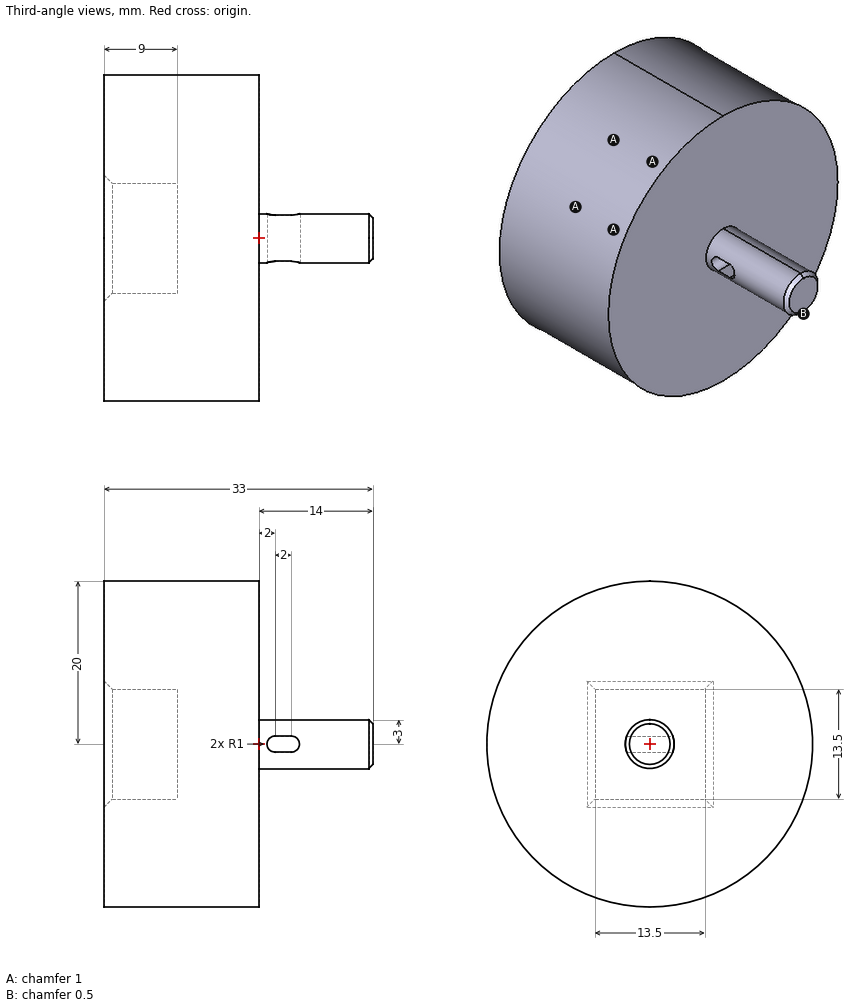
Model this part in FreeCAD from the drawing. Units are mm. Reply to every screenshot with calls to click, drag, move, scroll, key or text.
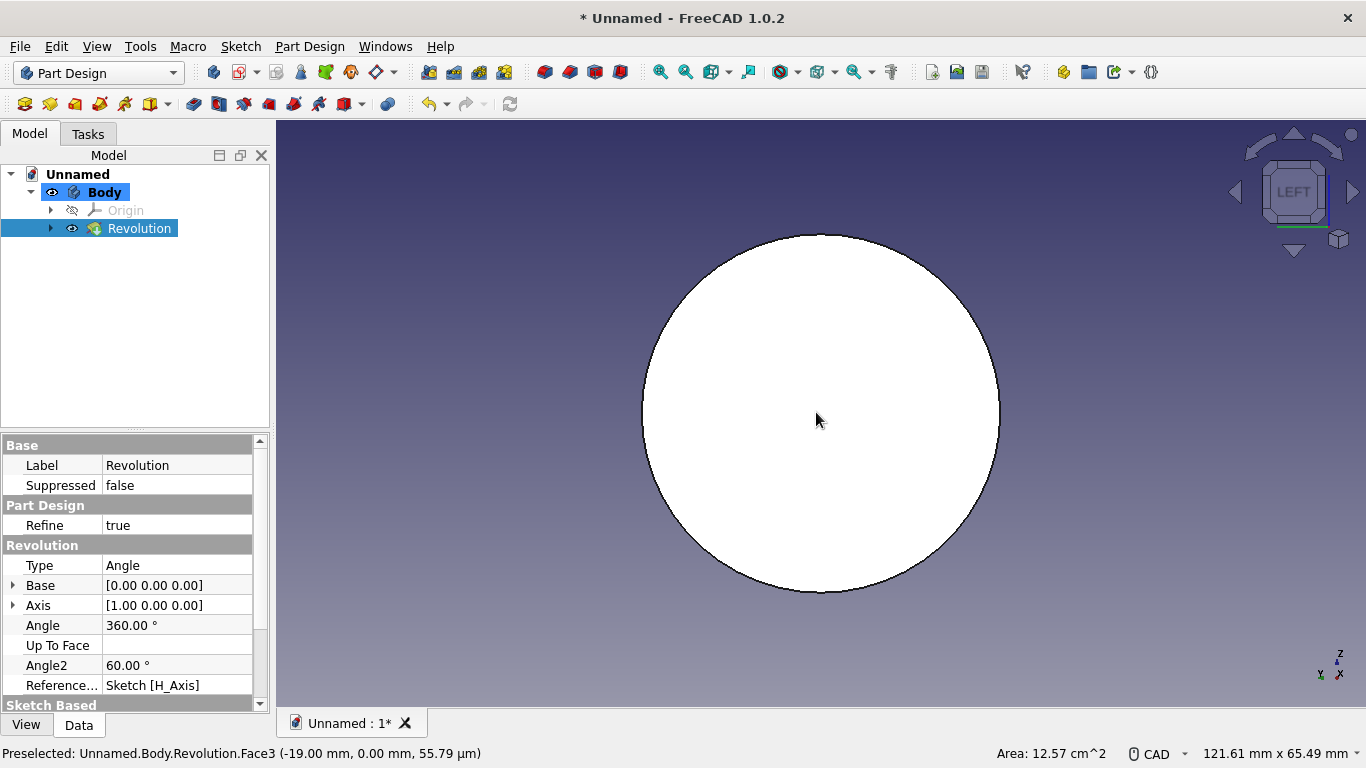
click(238, 72)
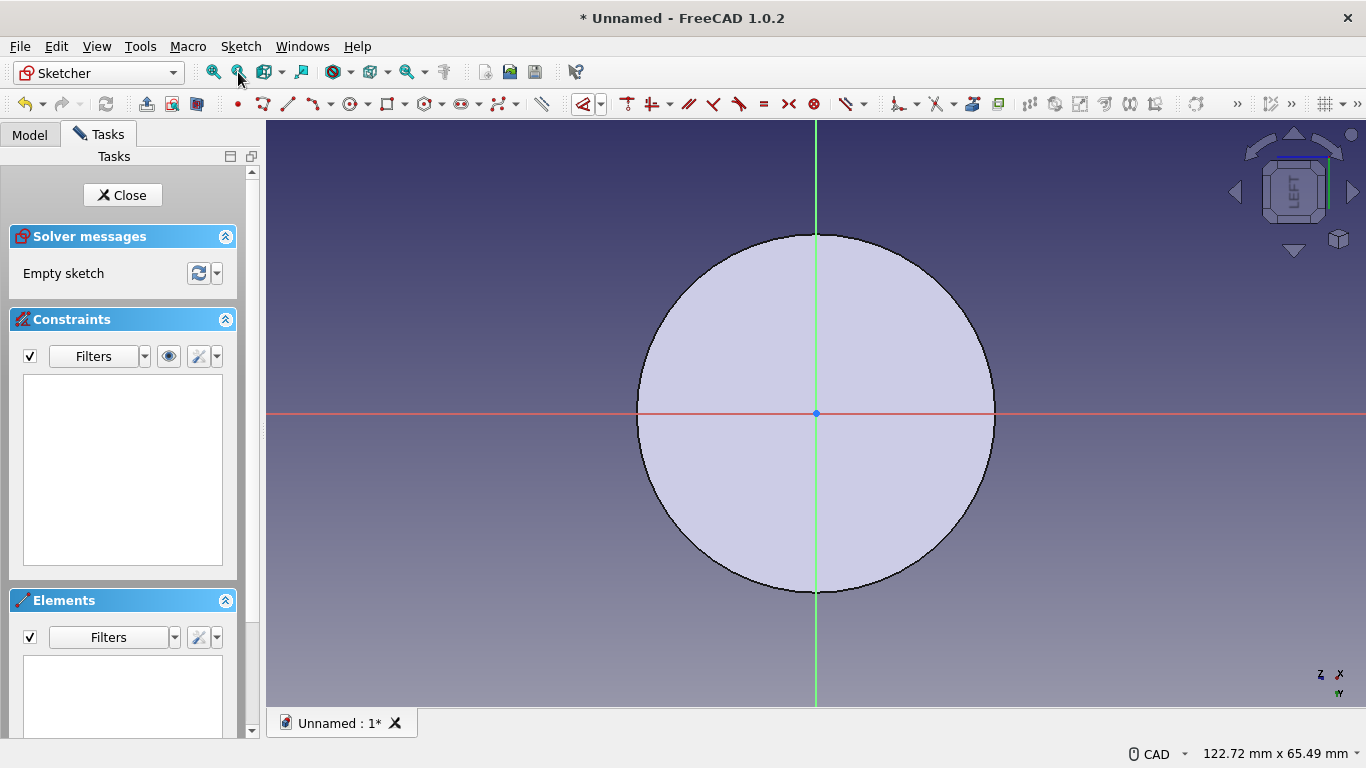
scroll(846, 414, up, 6)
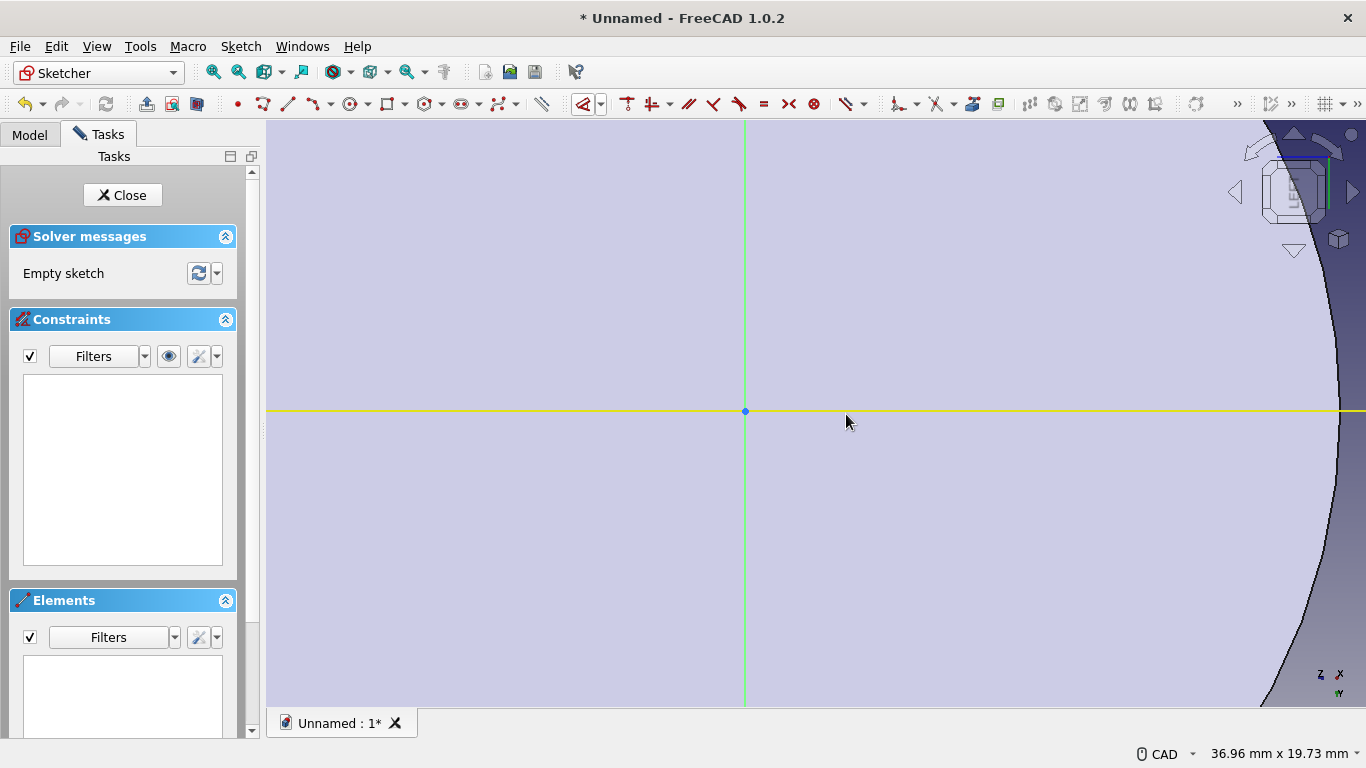
click(404, 104)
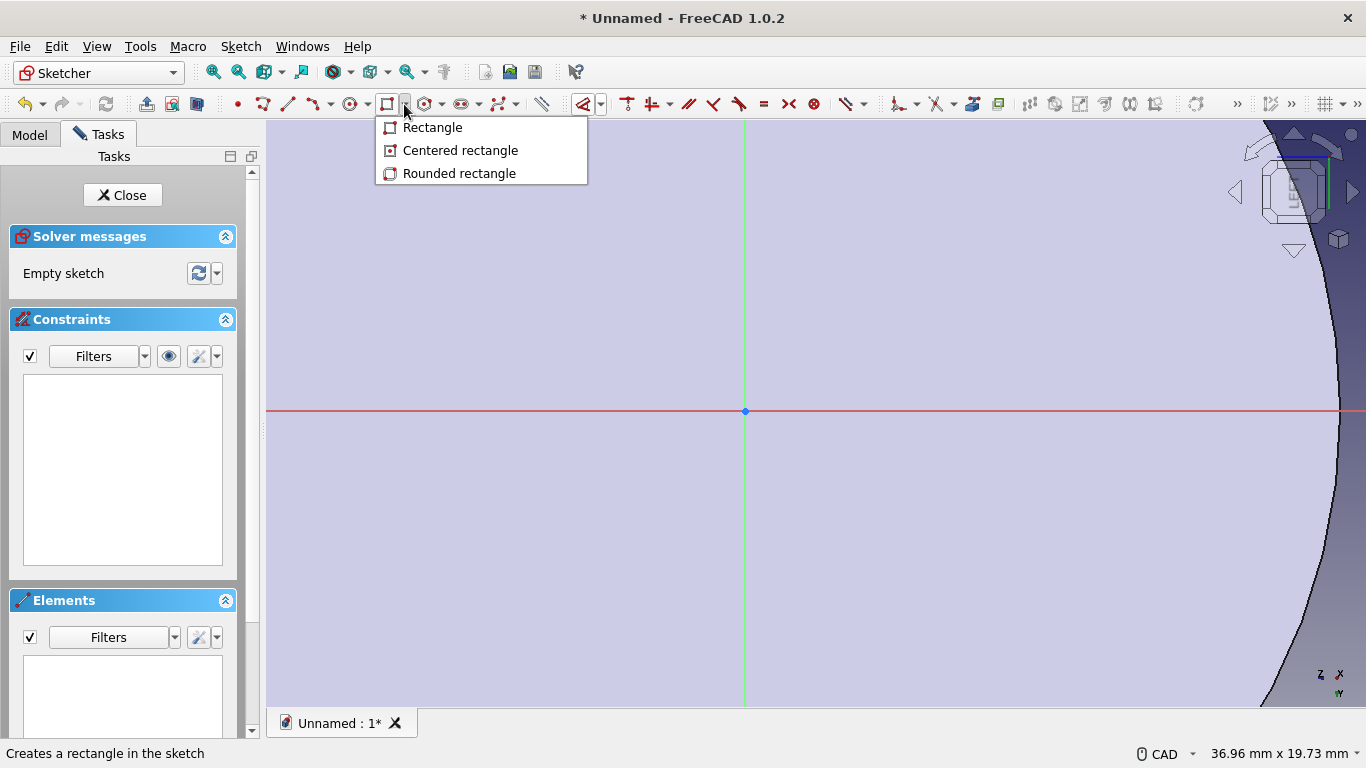
click(482, 150)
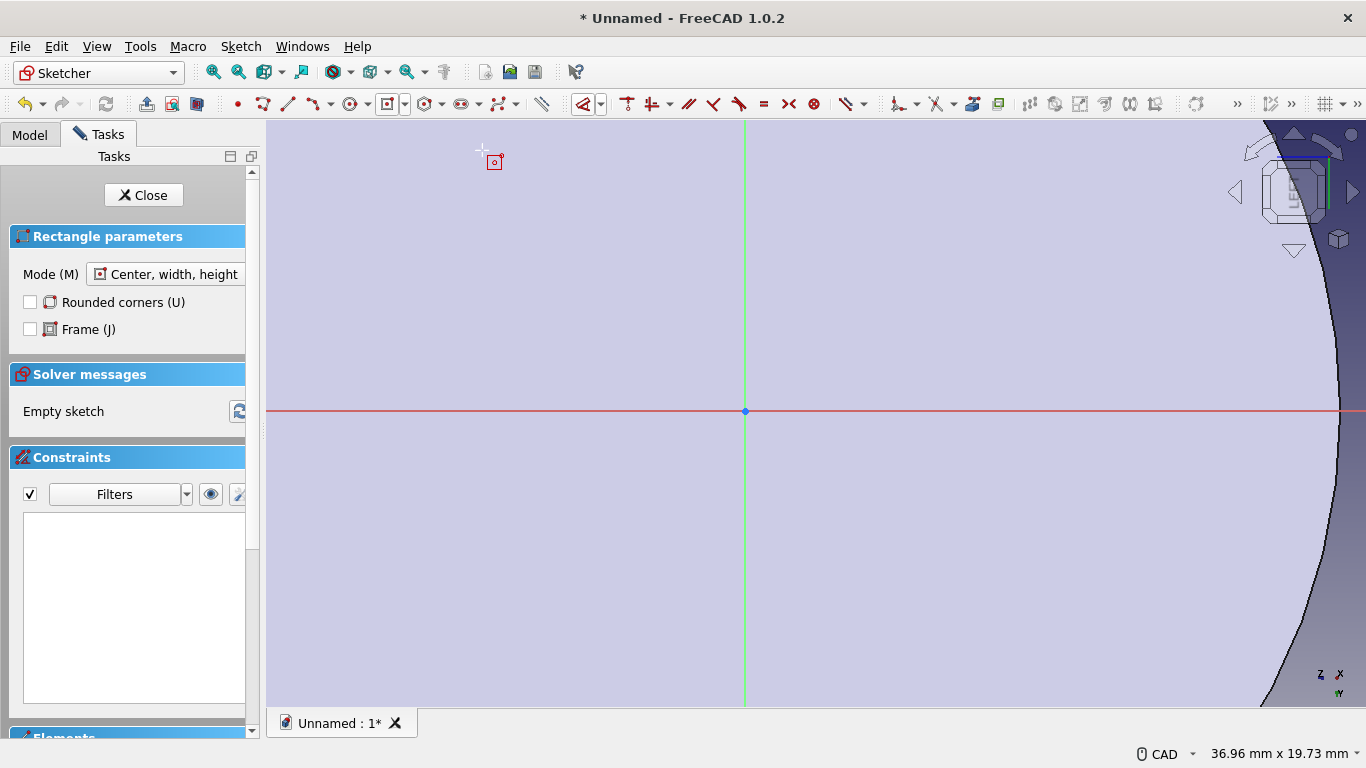
click(745, 411)
click(946, 210)
key(Escape)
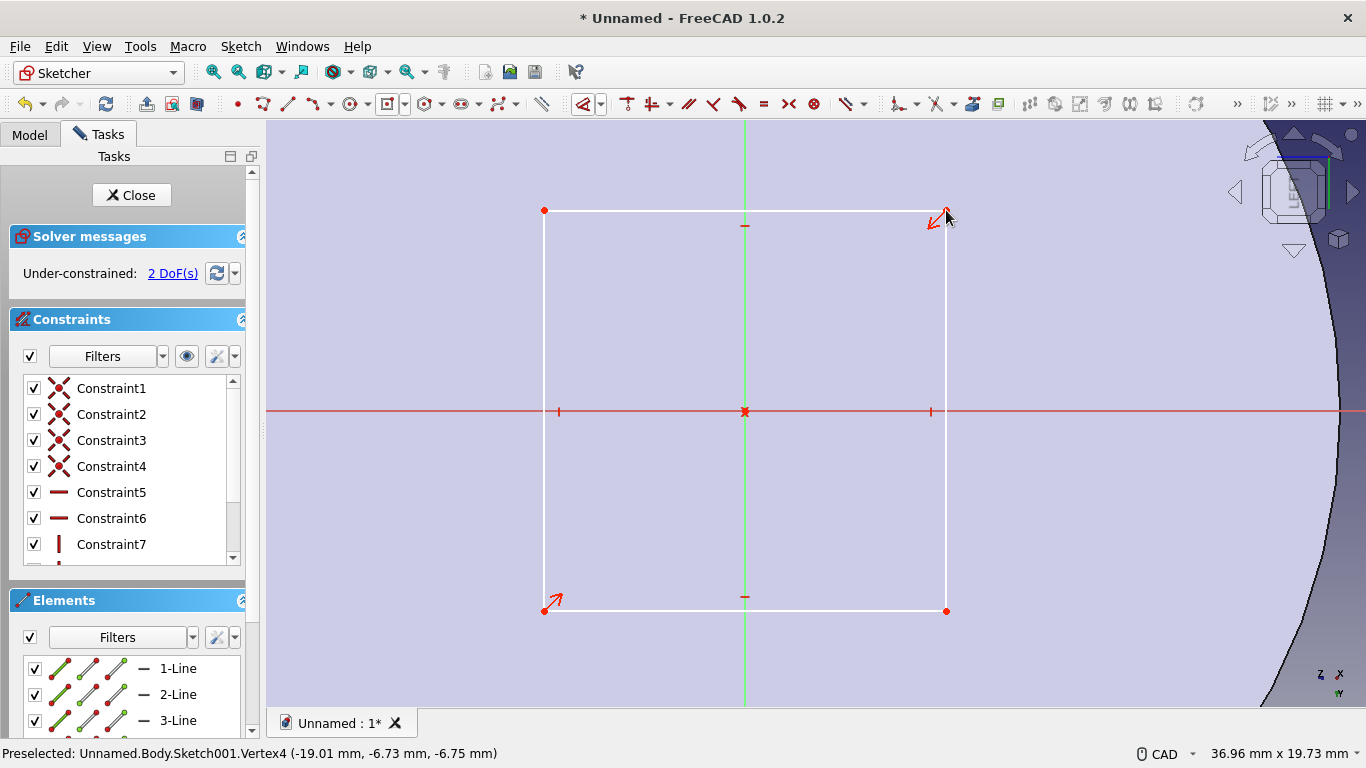
click(665, 611)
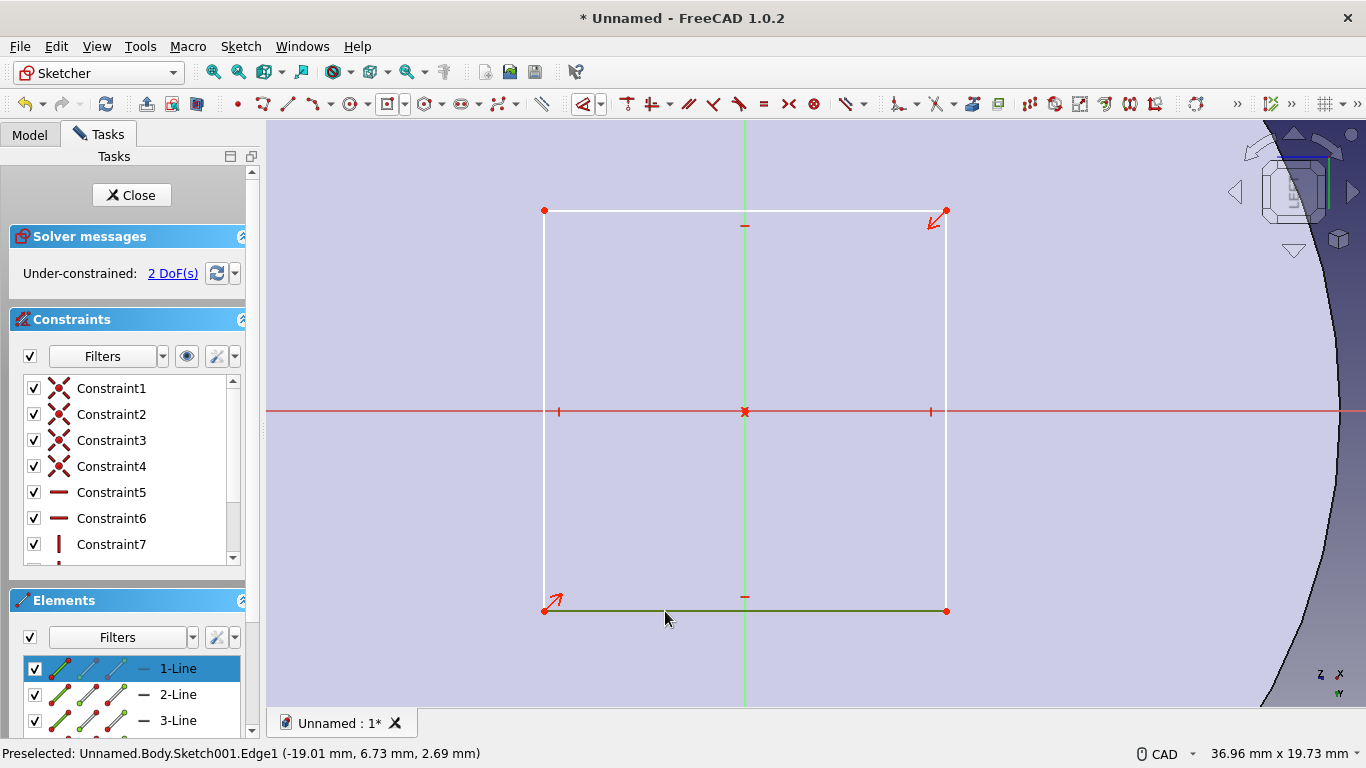
key(l)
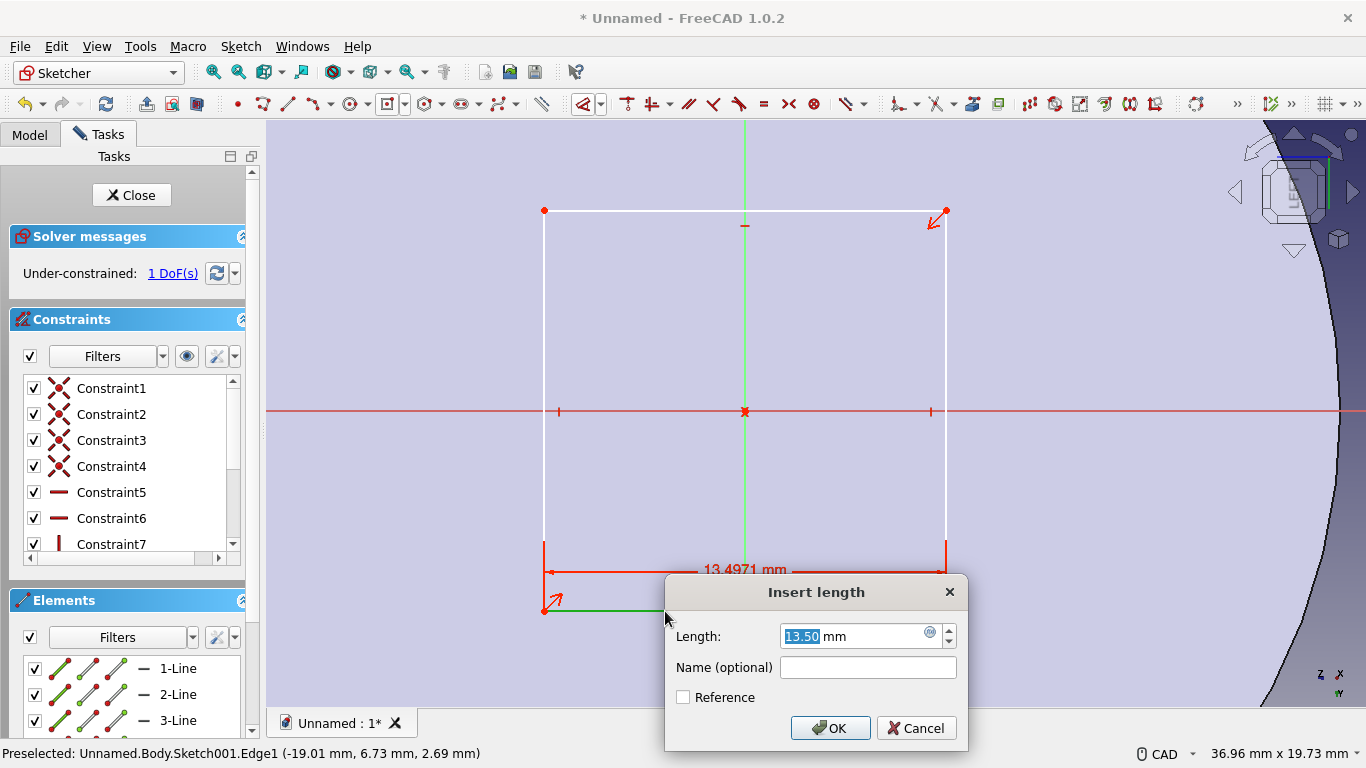
text(13.5)
key(Return)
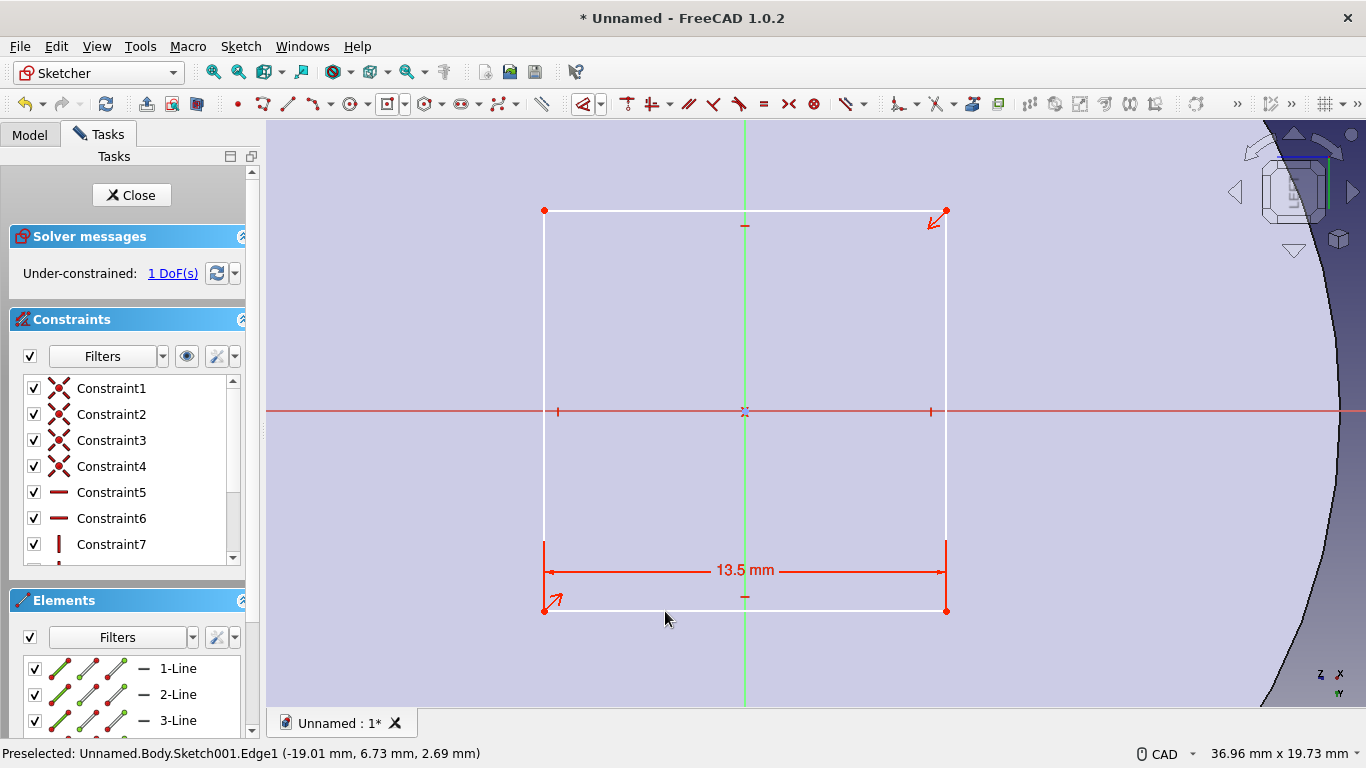
click(946, 491)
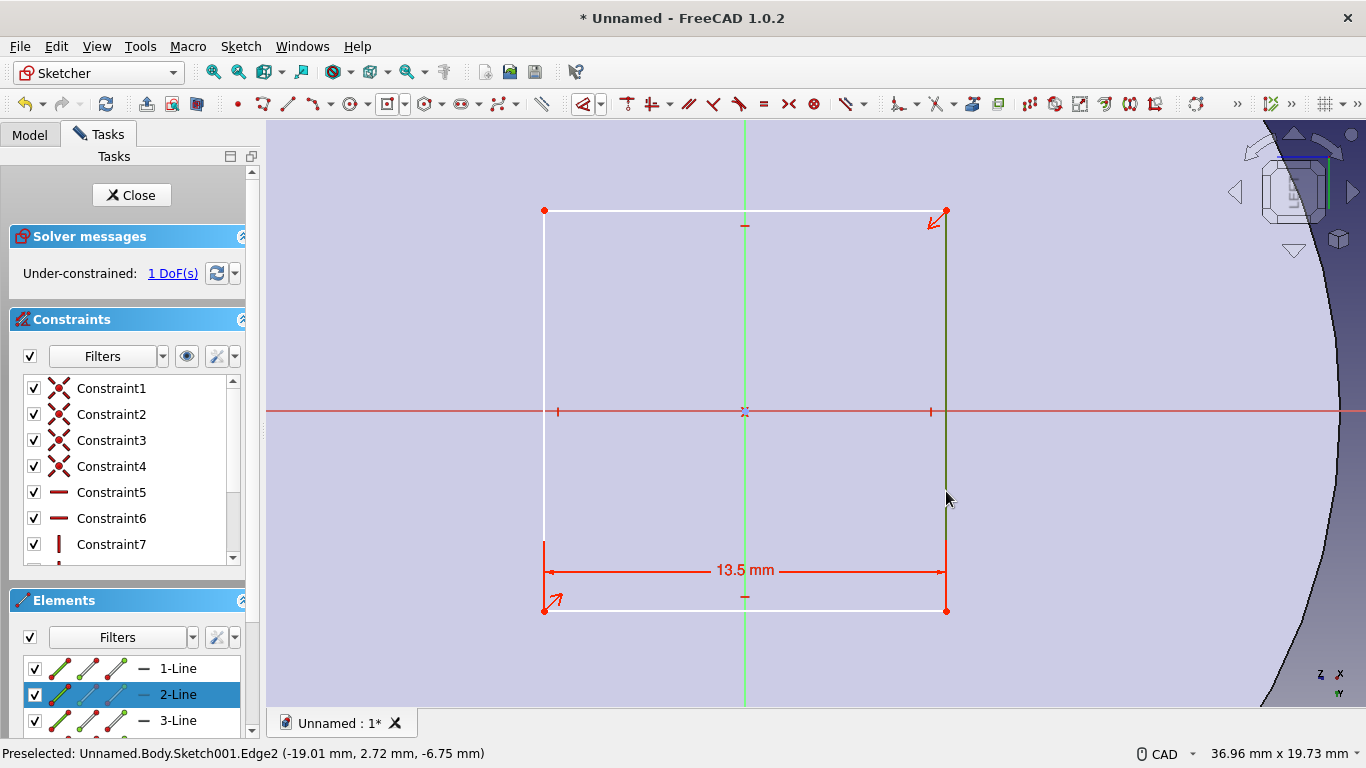
key(i)